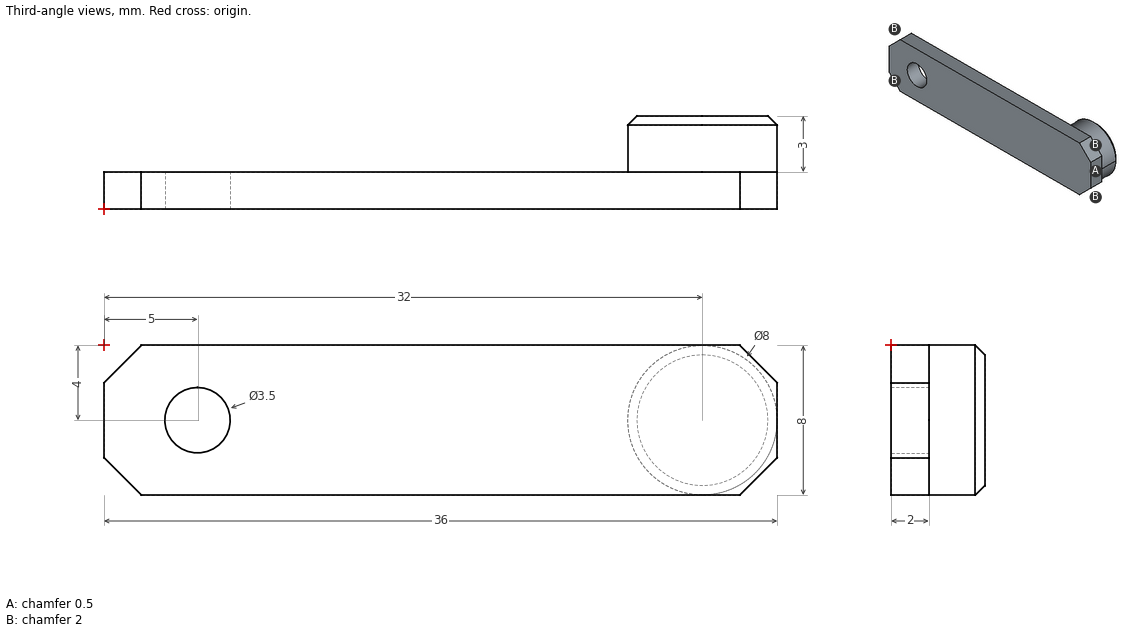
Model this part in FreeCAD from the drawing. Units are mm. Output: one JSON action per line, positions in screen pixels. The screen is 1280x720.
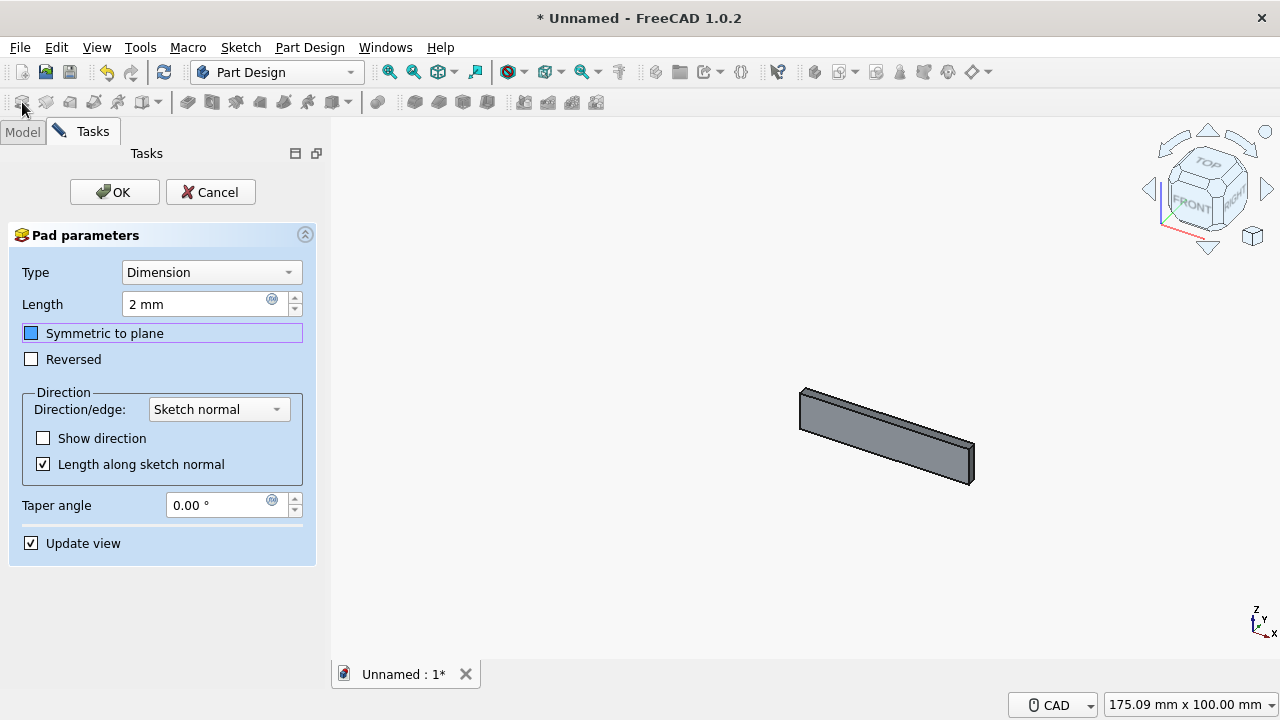
{"action": "left_click", "coordinate": [30, 359]}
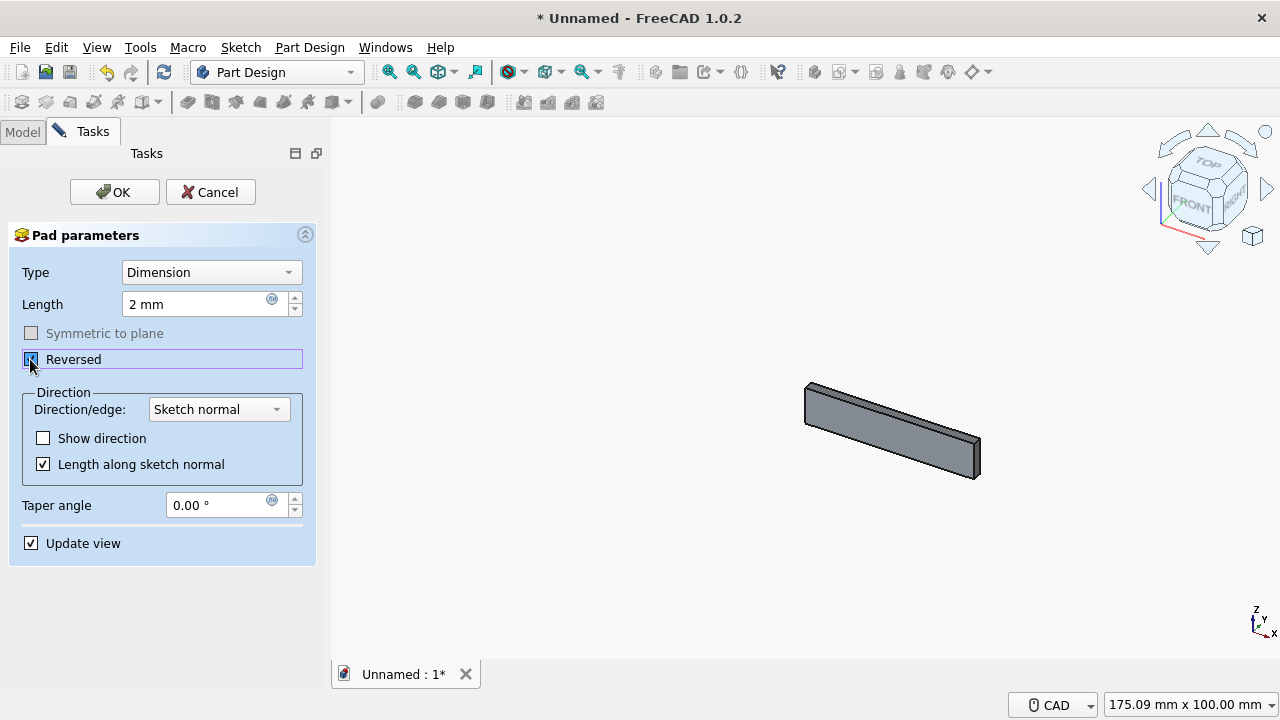
{"action": "left_click", "coordinate": [115, 192]}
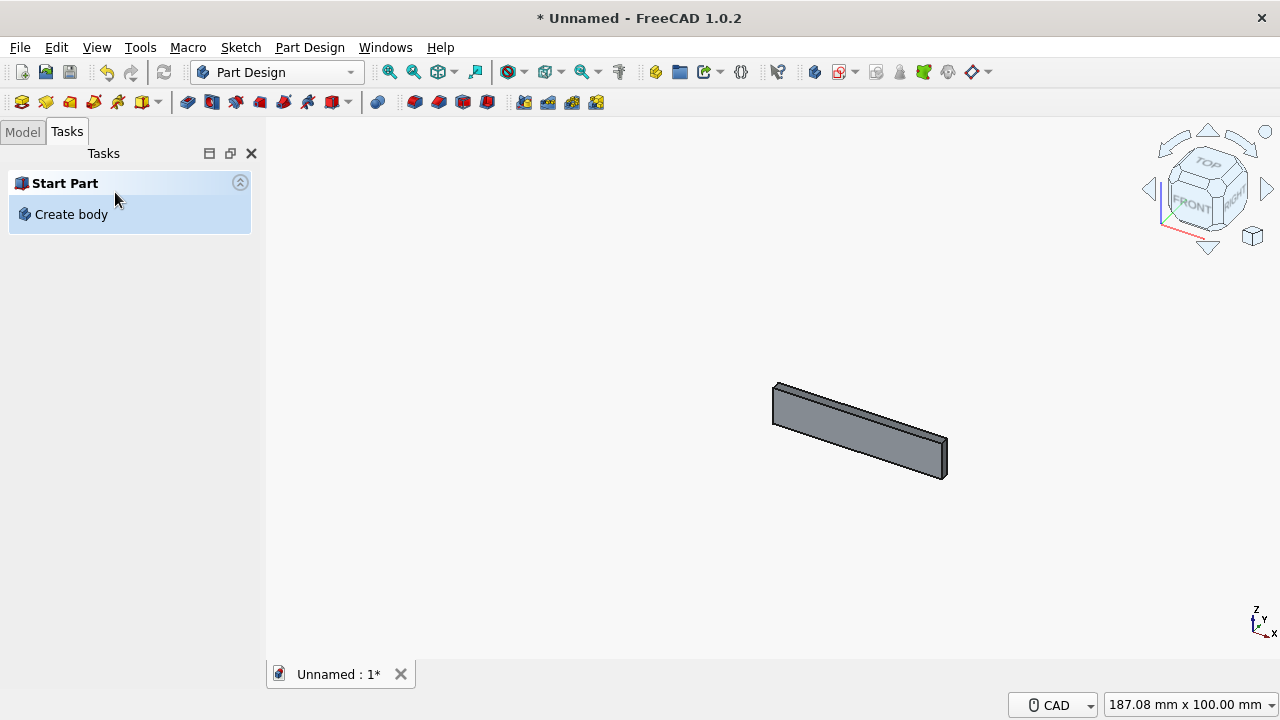
{"action": "key", "text": "v f"}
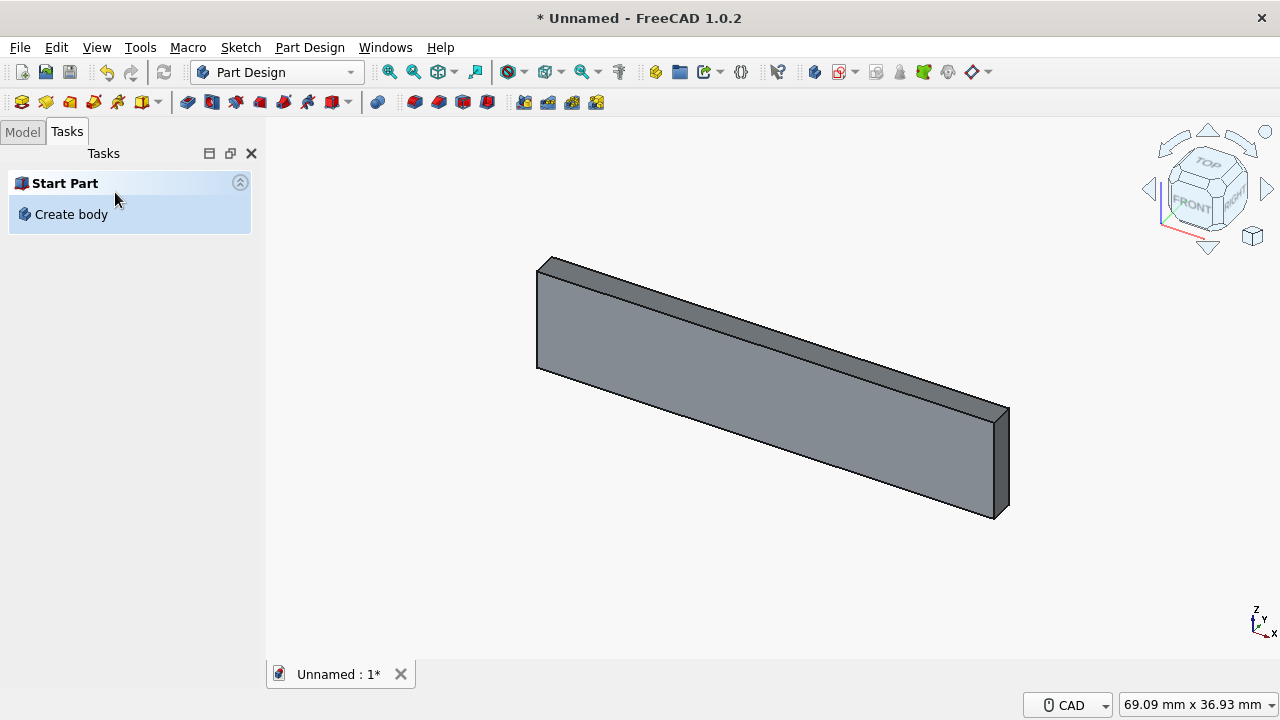
{"action": "key", "text": "4"}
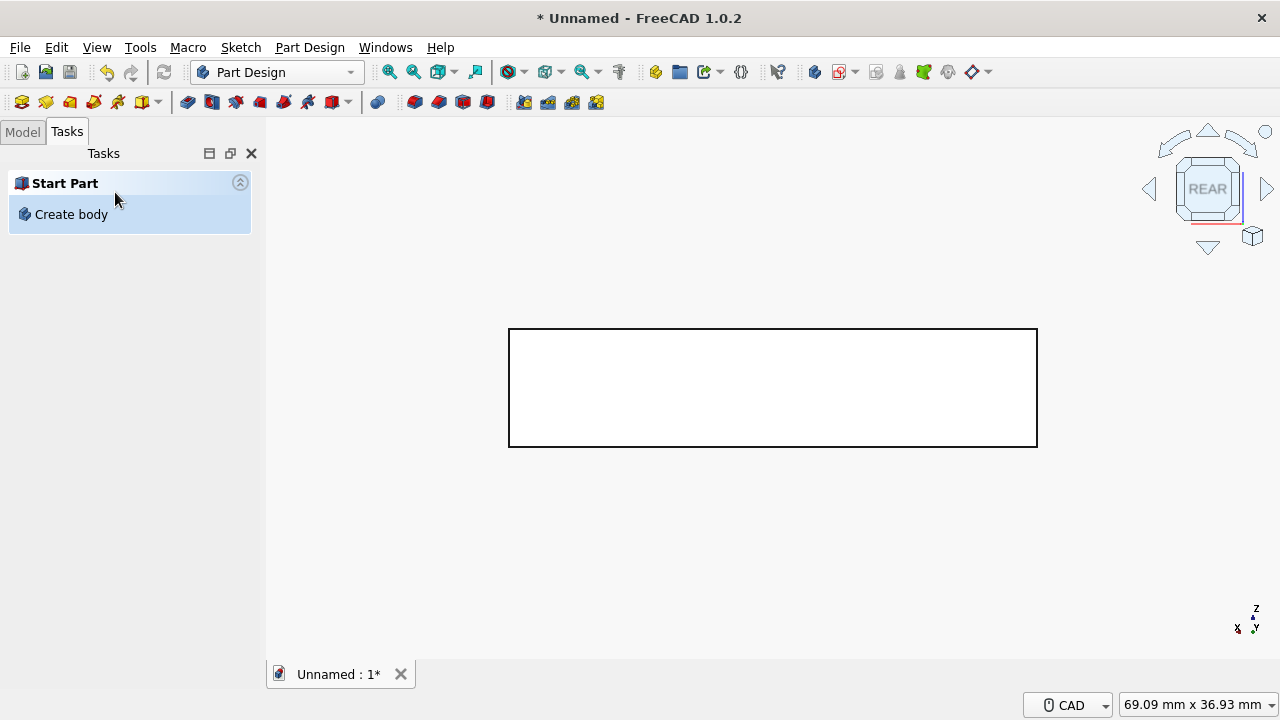
{"action": "left_click", "coordinate": [622, 387]}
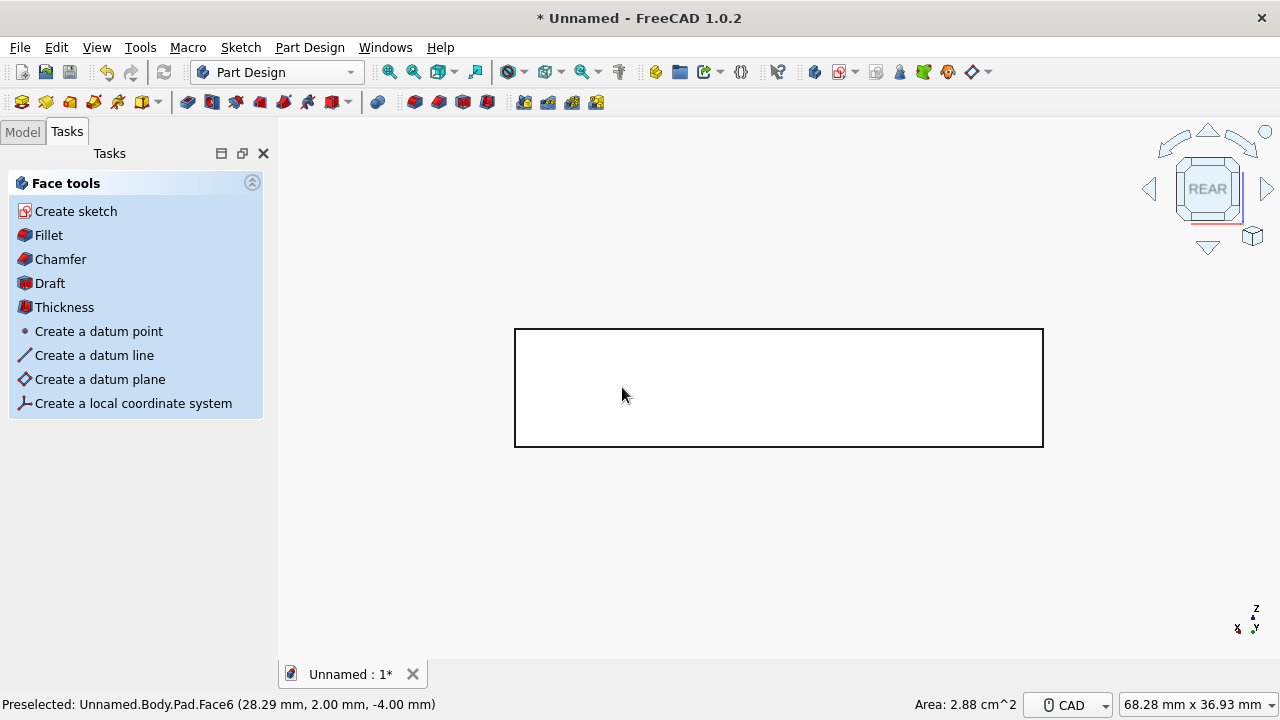
{"action": "left_click", "coordinate": [840, 72]}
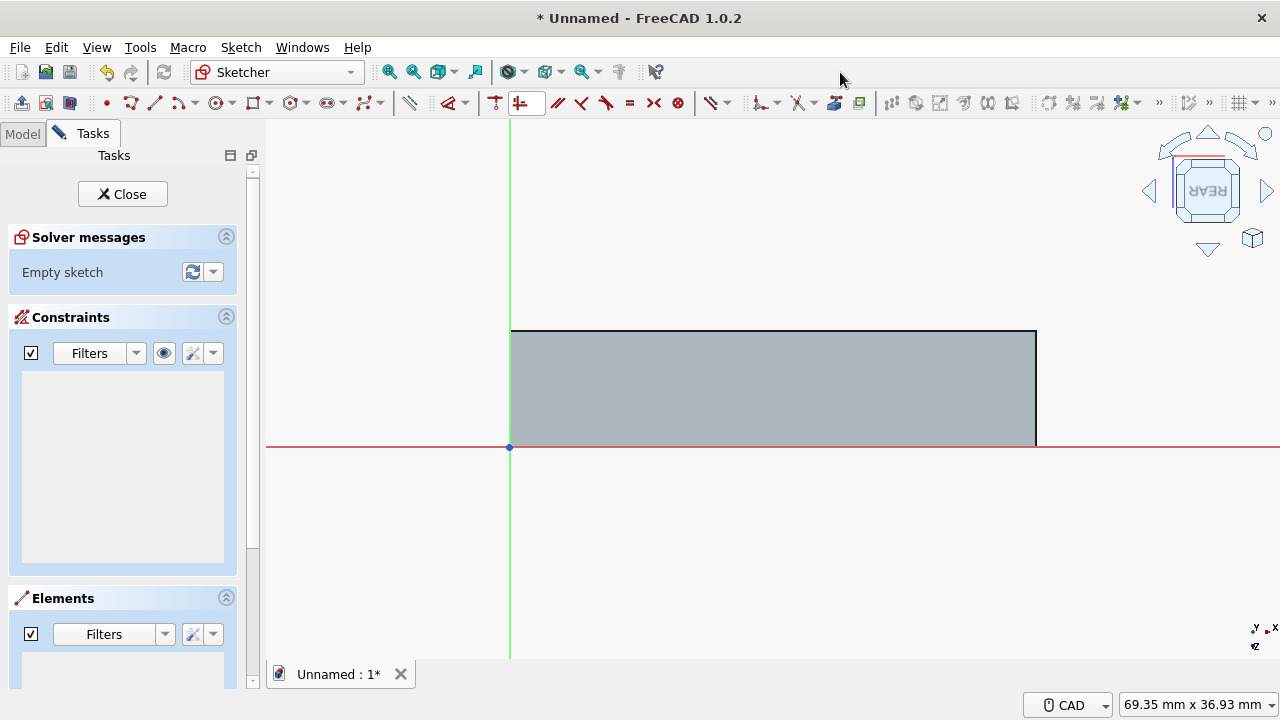
{"action": "scroll", "coordinate": [512, 411], "scroll_direction": "up", "scroll_amount": 7}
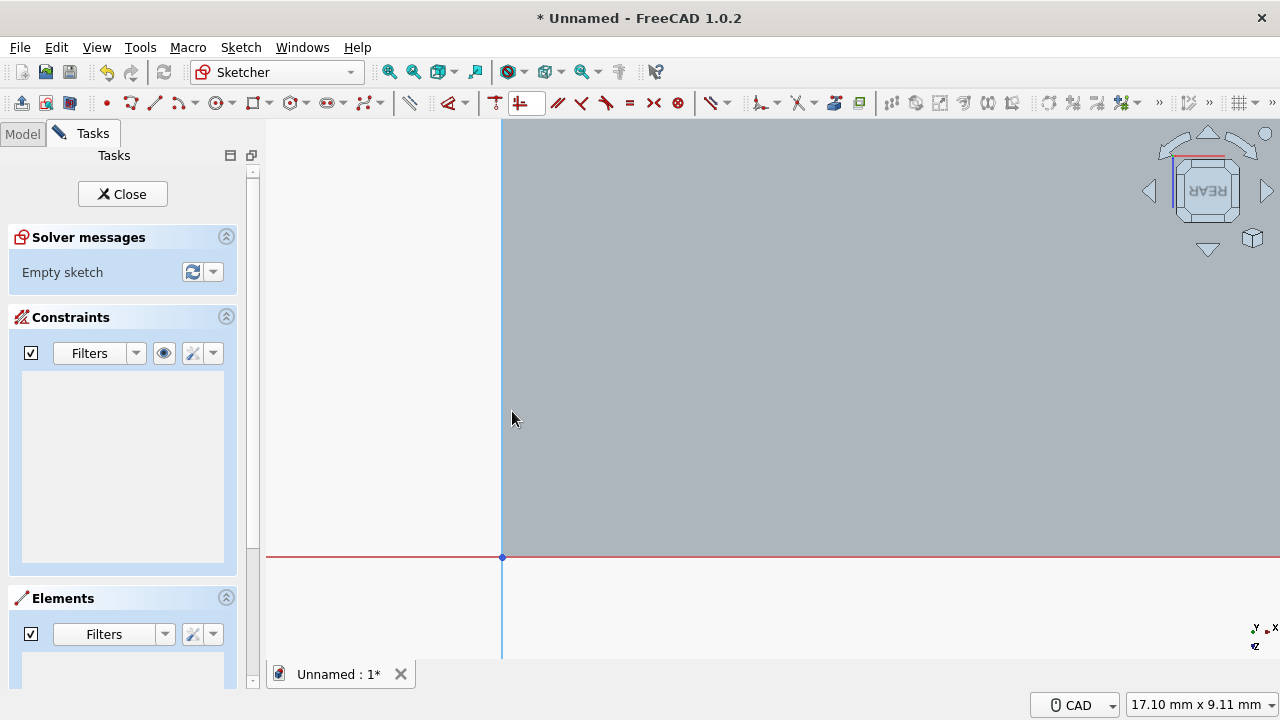
{"action": "left_click", "coordinate": [216, 104]}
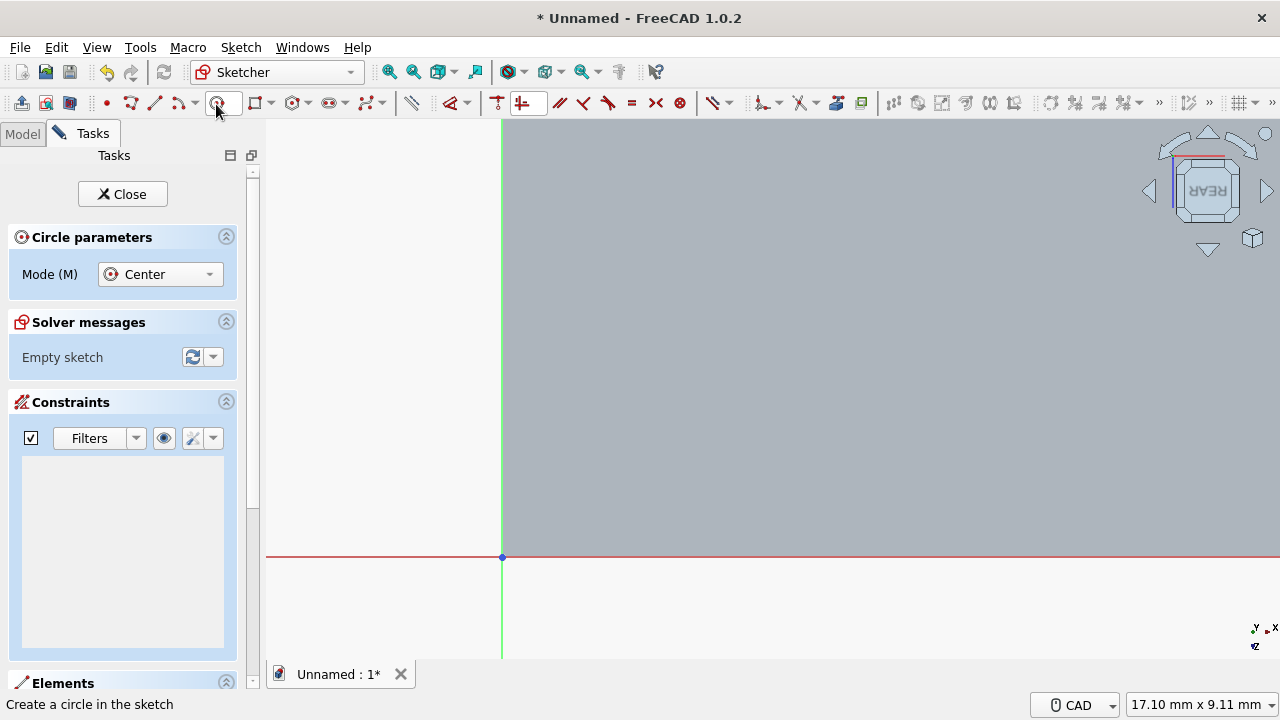
{"action": "left_click", "coordinate": [799, 320]}
{"action": "mouse_move", "coordinate": [872, 247]}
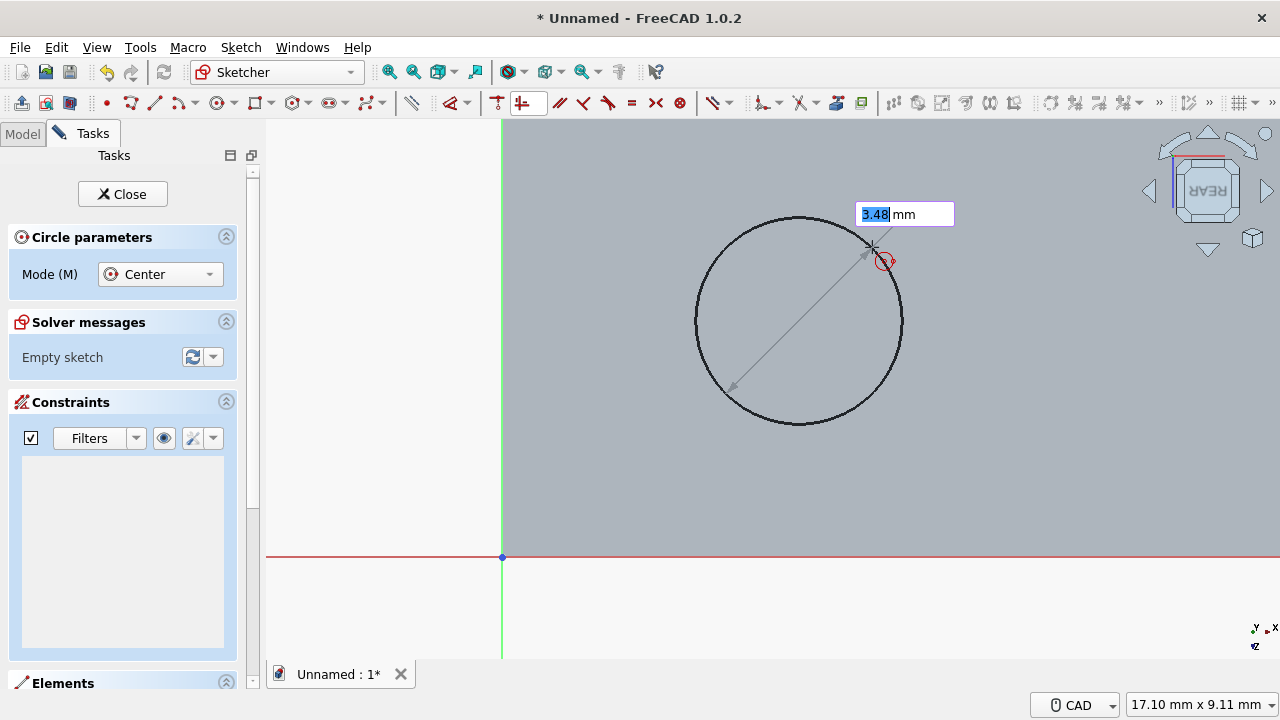
{"action": "type", "text": "3.5"}
{"action": "key", "text": "Return"}
{"action": "key", "text": "Escape"}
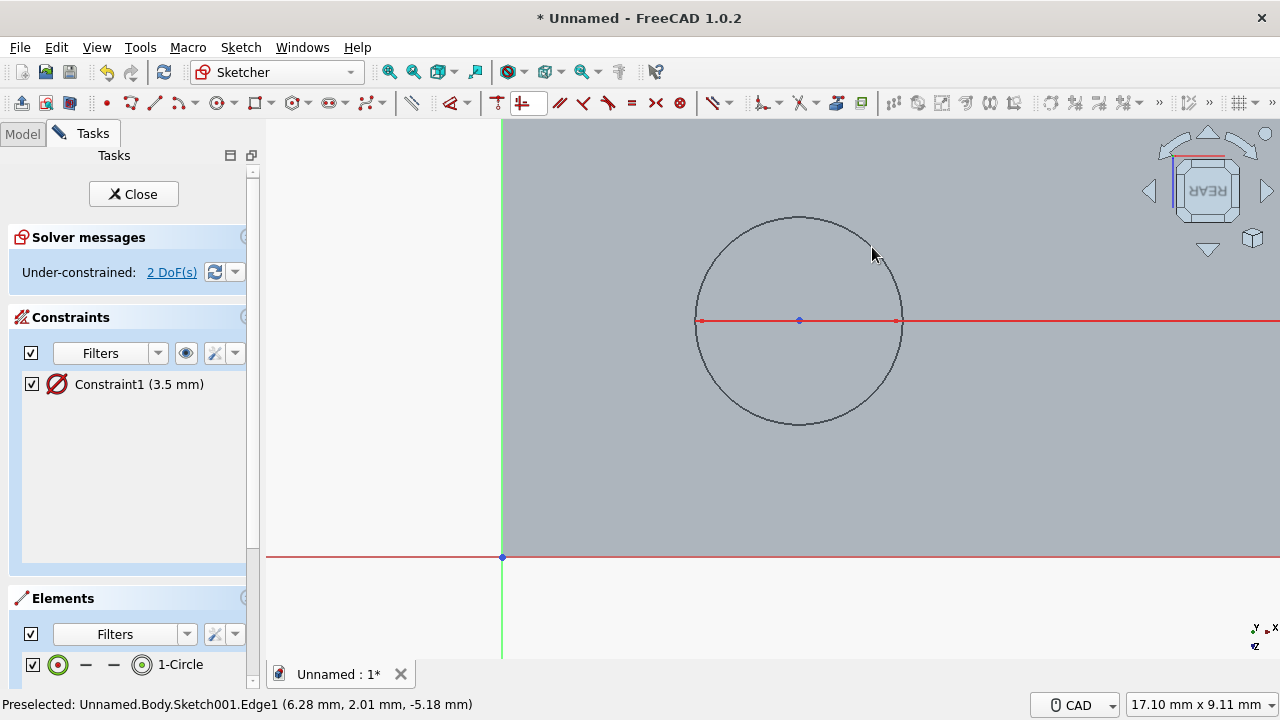
{"action": "key", "text": "d"}